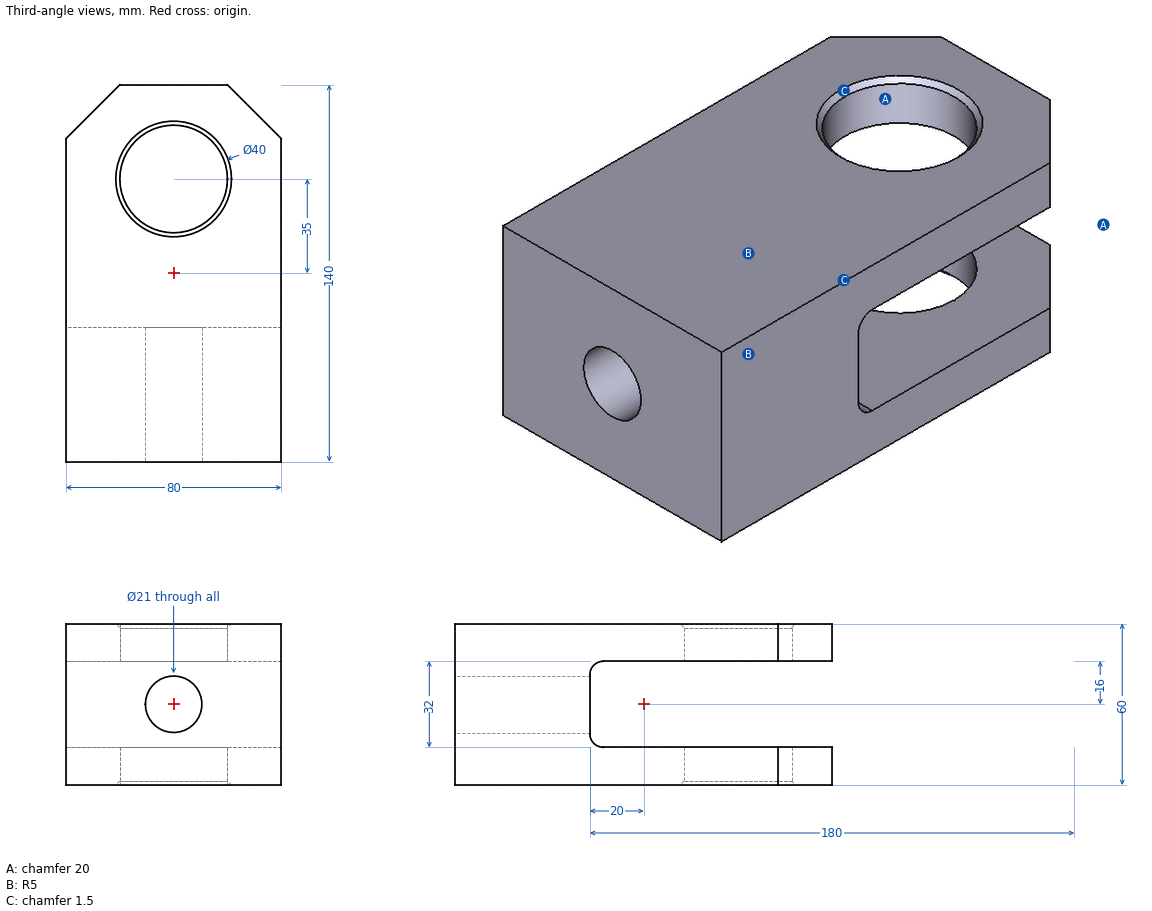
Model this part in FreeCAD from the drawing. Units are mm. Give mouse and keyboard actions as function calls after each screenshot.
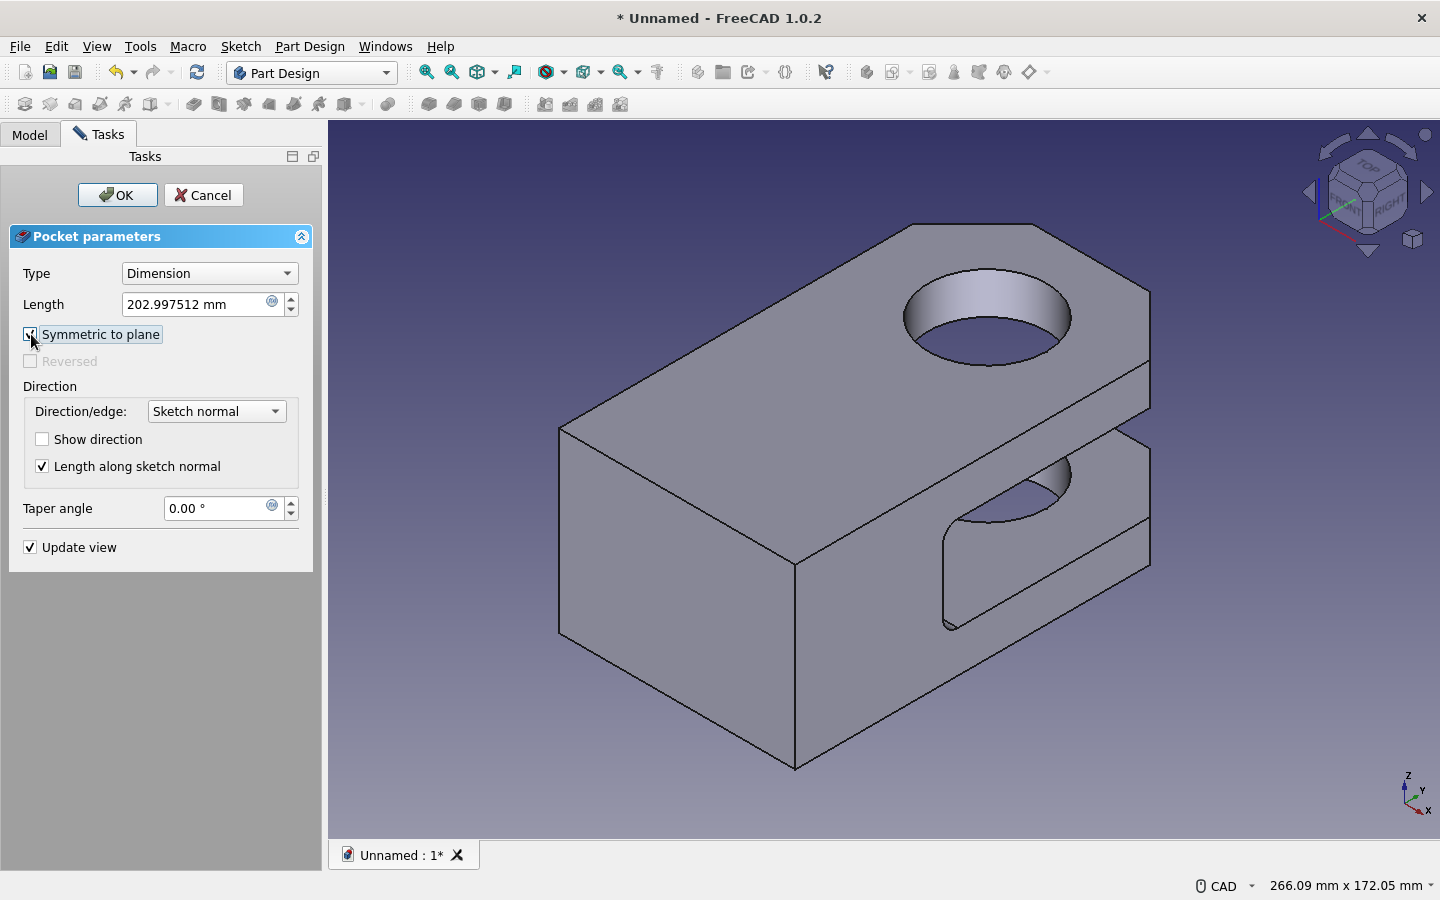
click(118, 195)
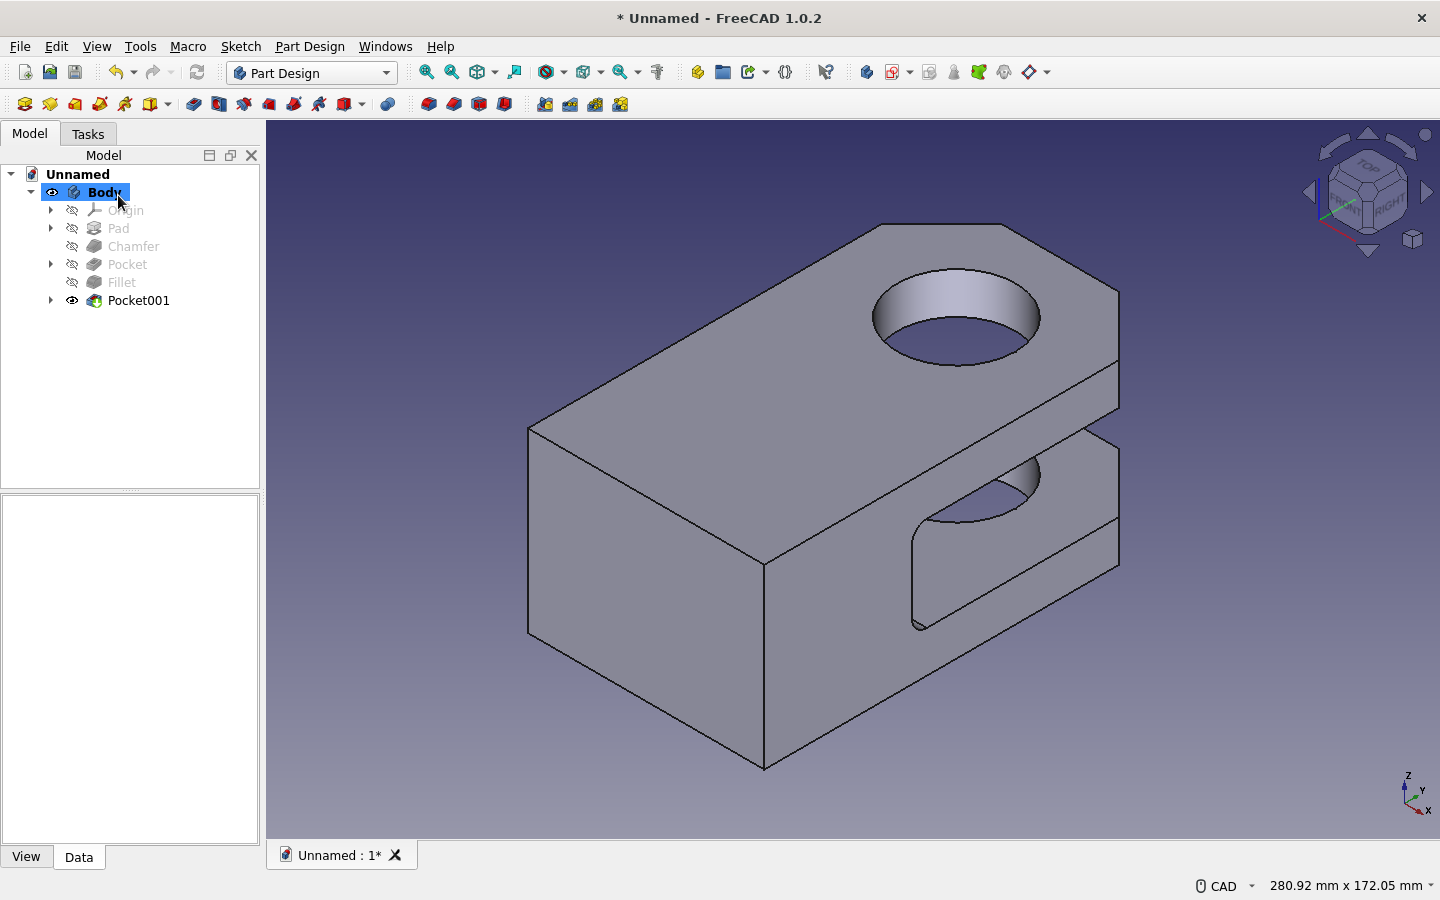
click(897, 282)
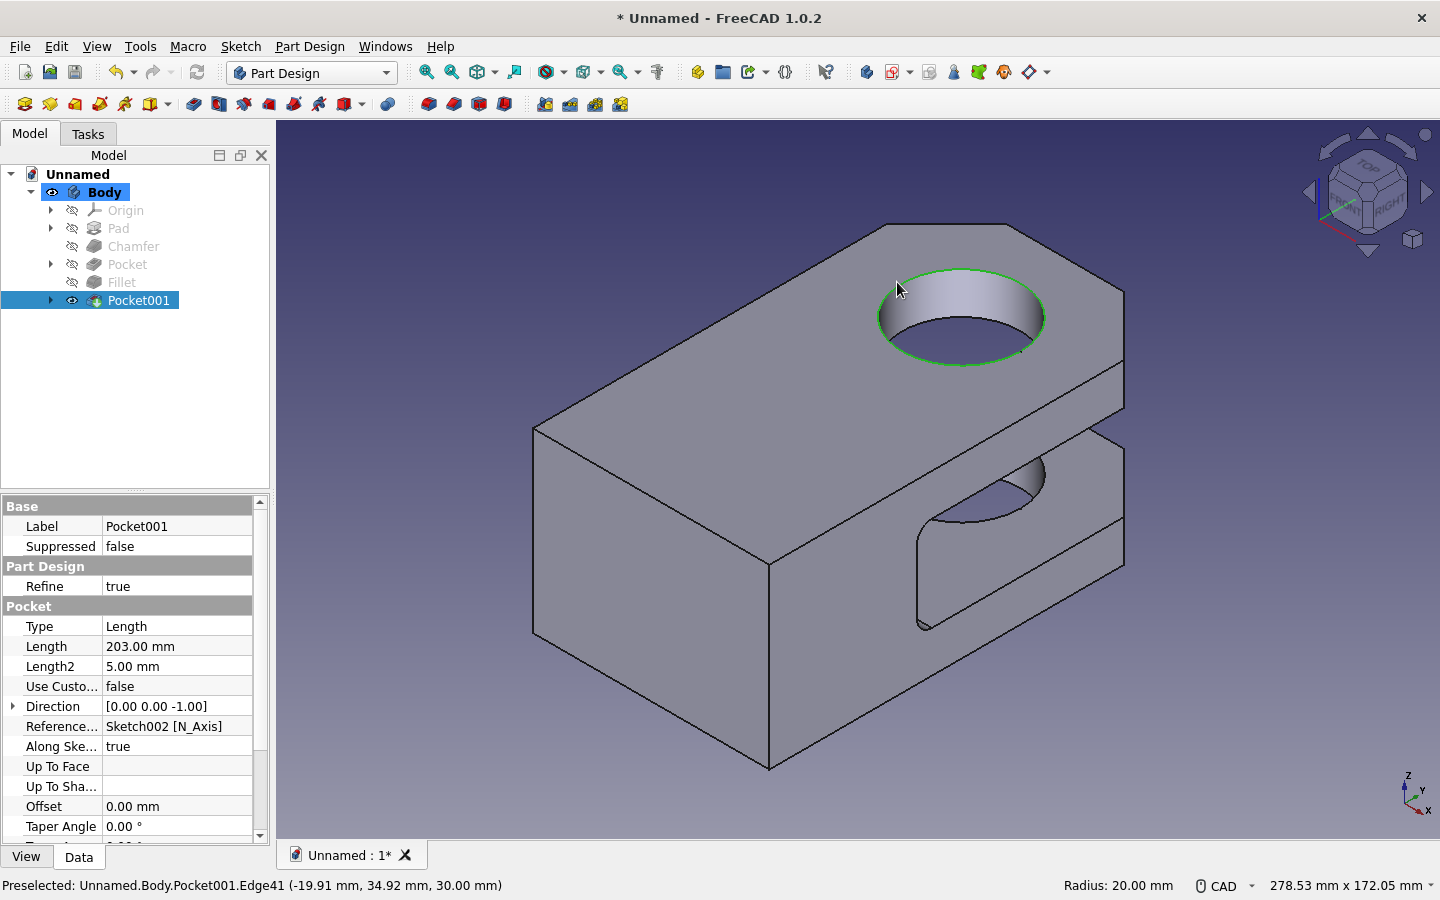
key(2)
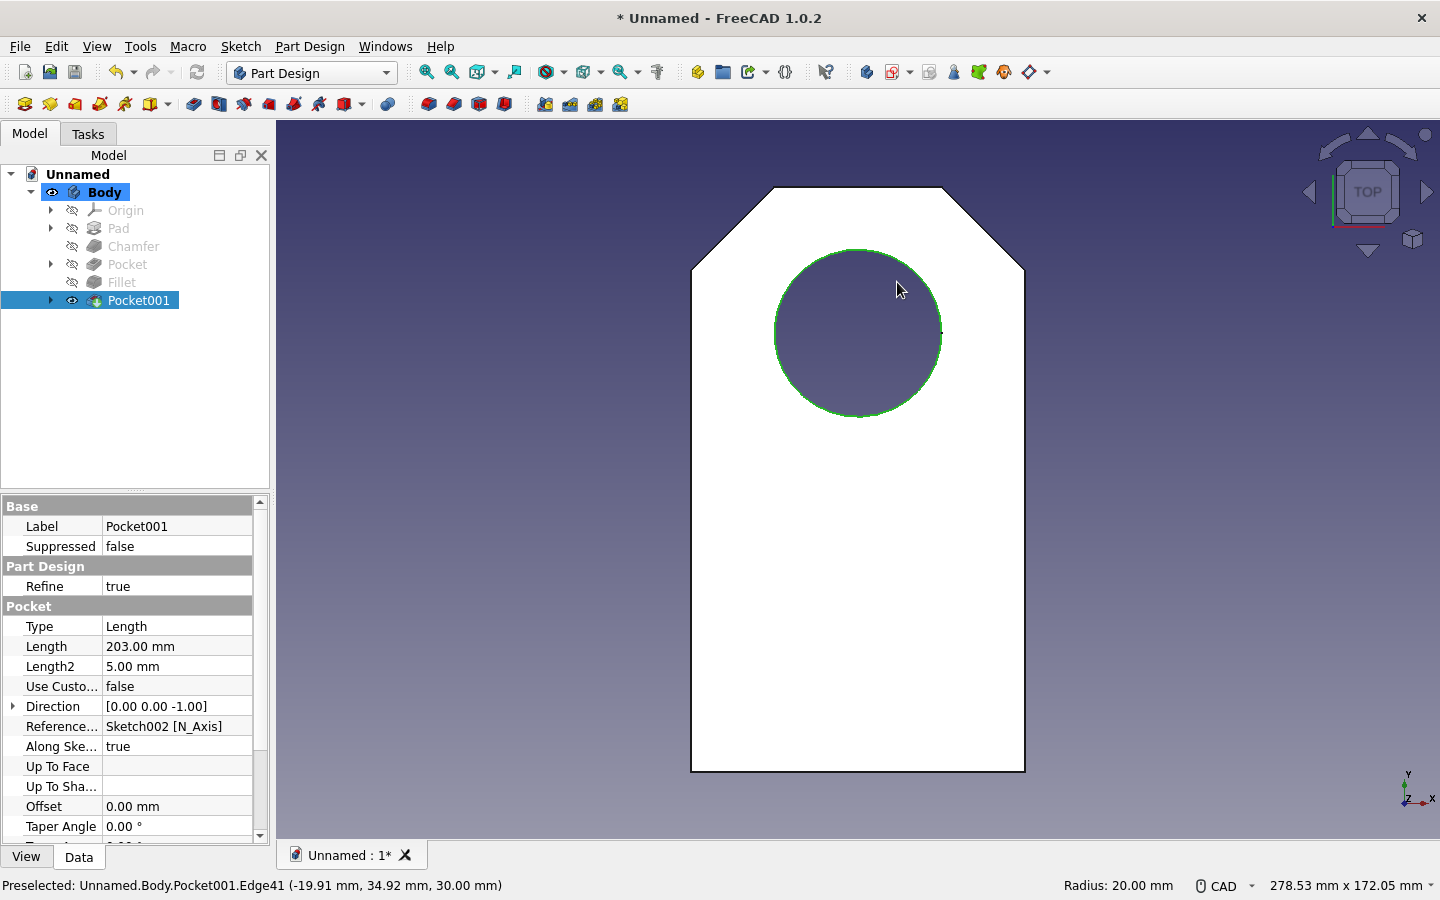
key(0)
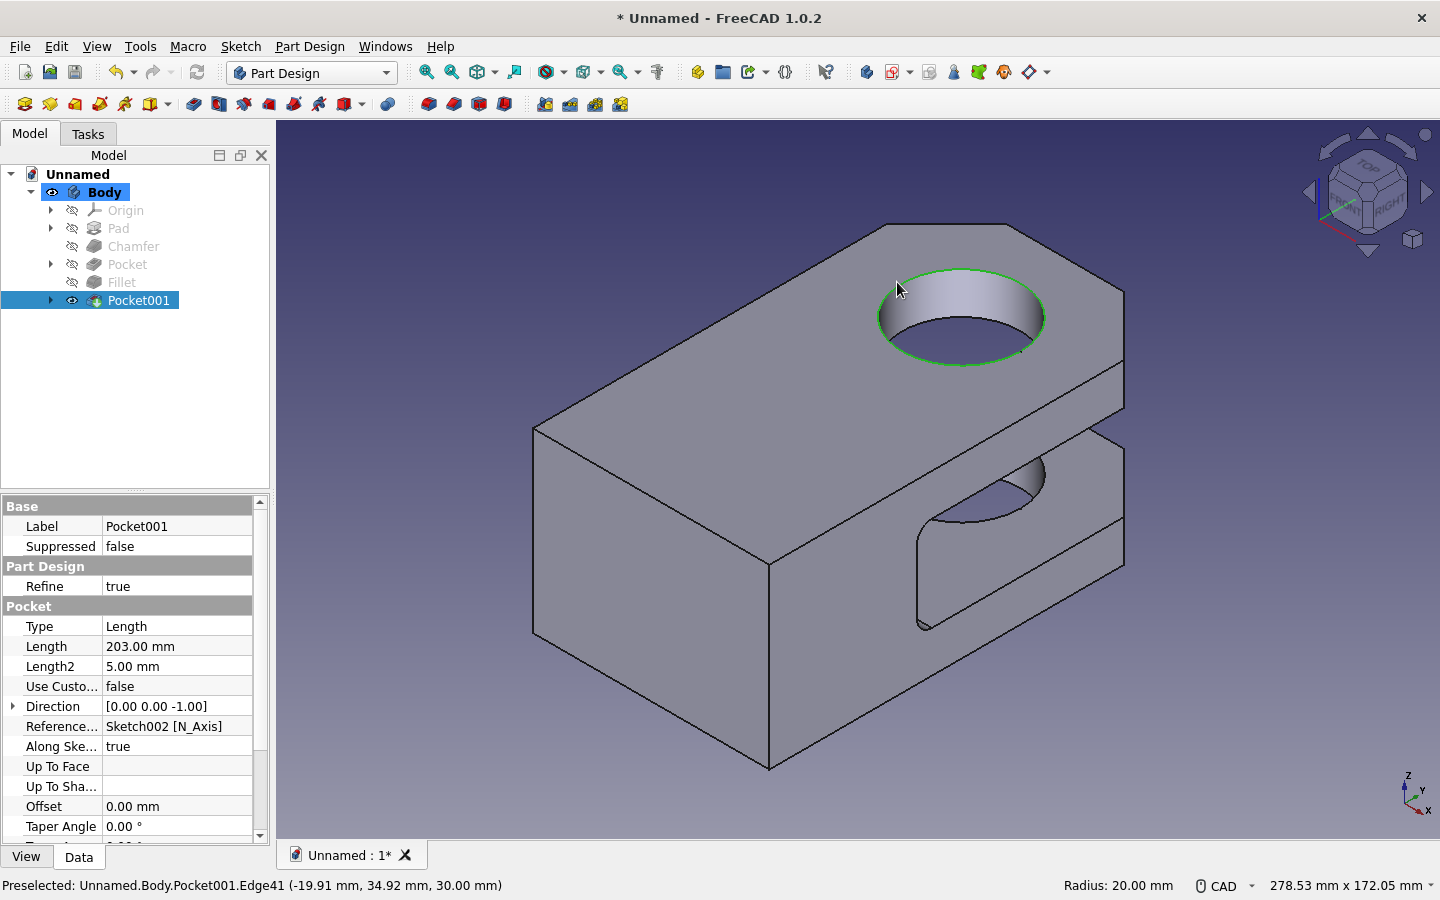
key(1)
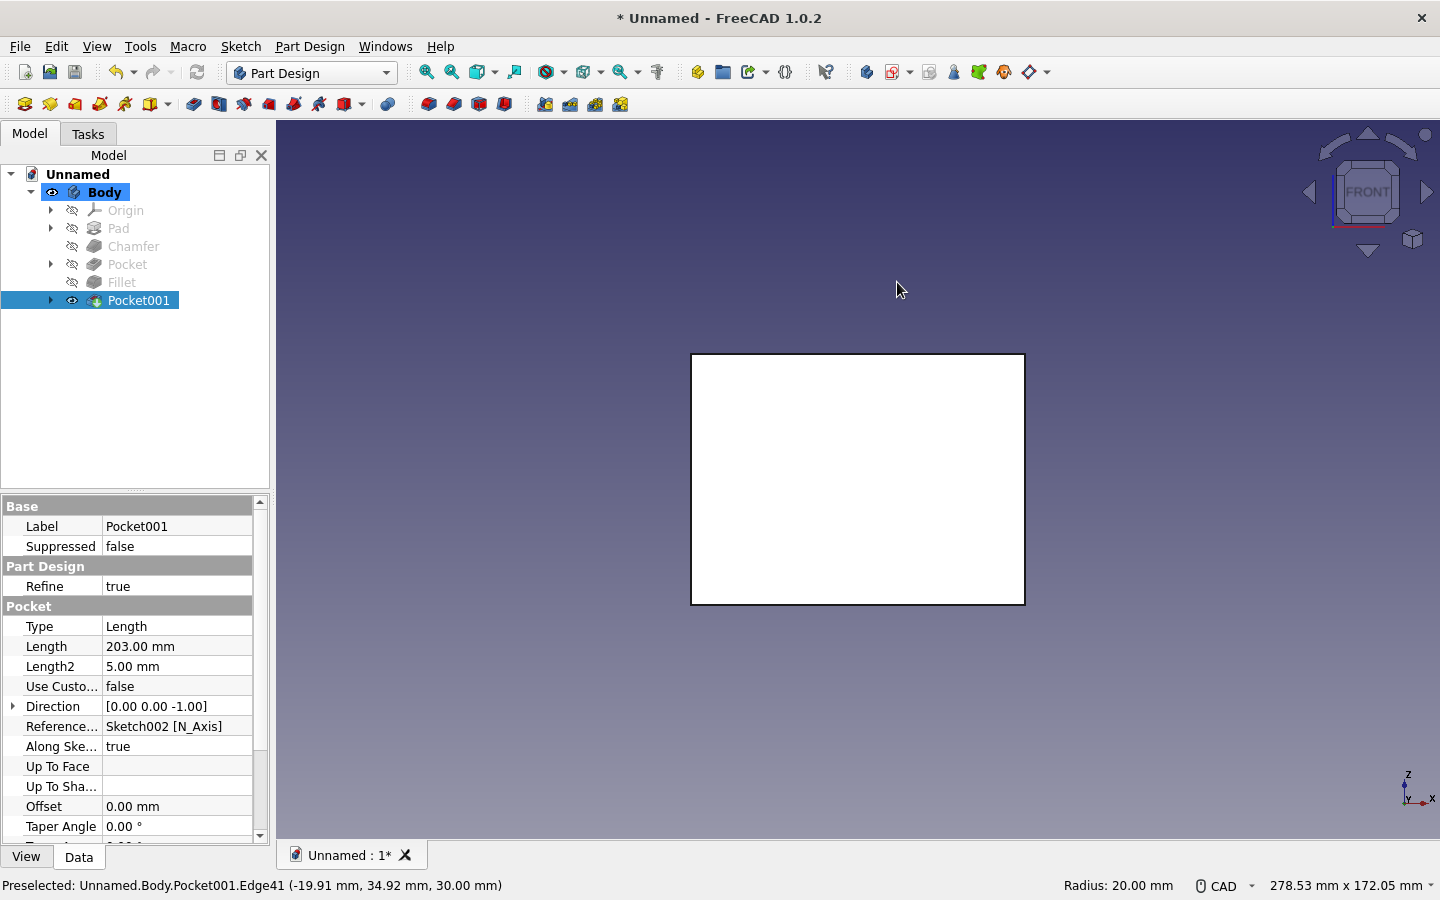
key(v)
key(f)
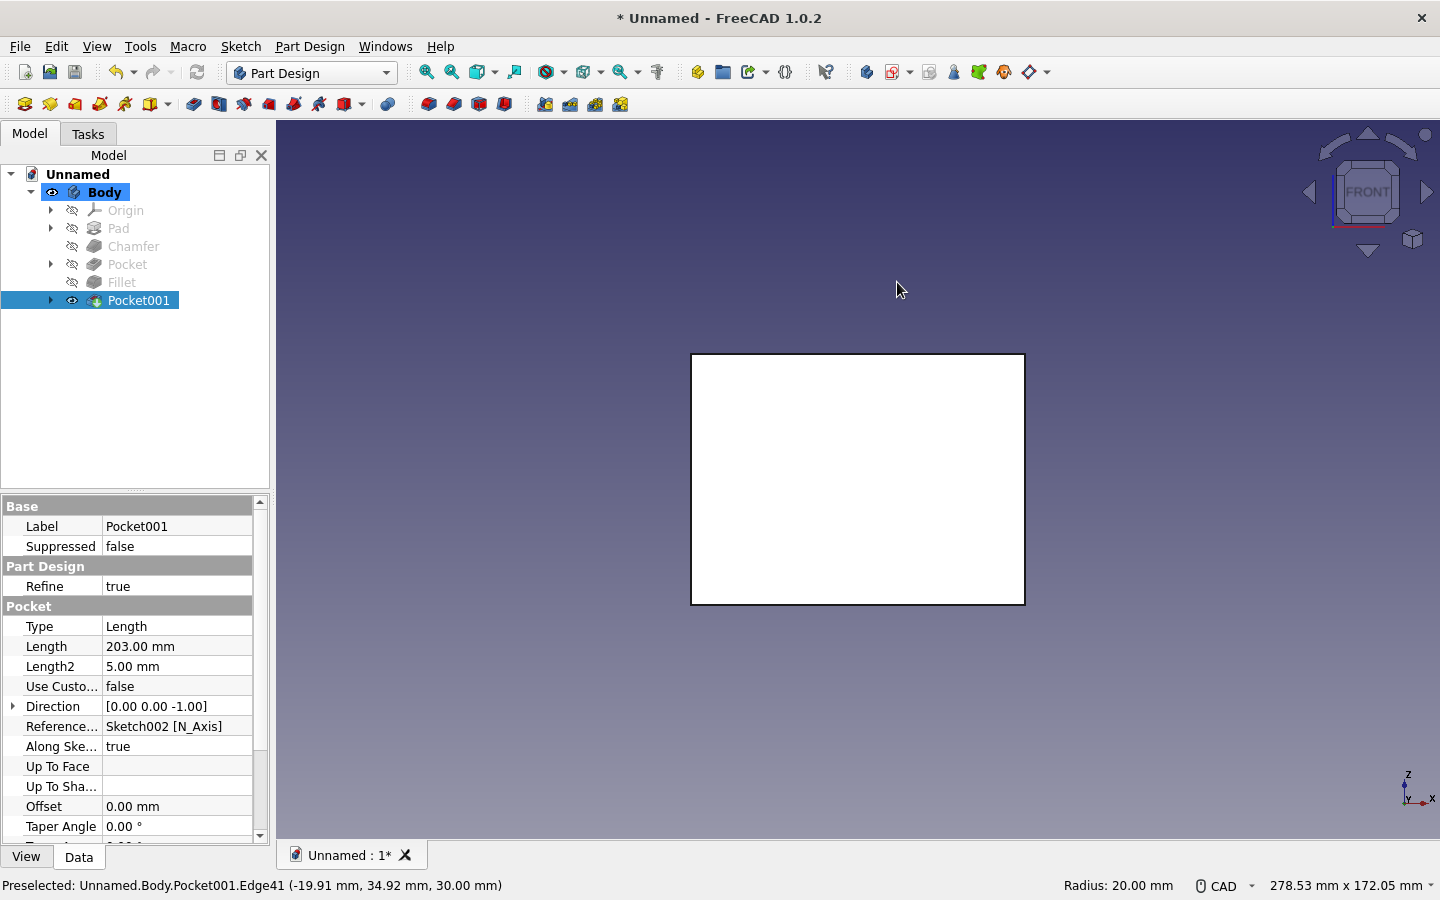
key(3)